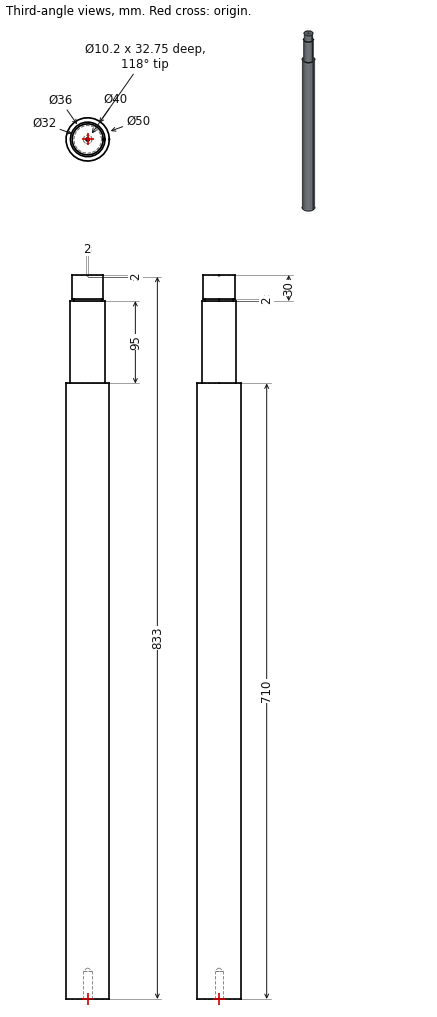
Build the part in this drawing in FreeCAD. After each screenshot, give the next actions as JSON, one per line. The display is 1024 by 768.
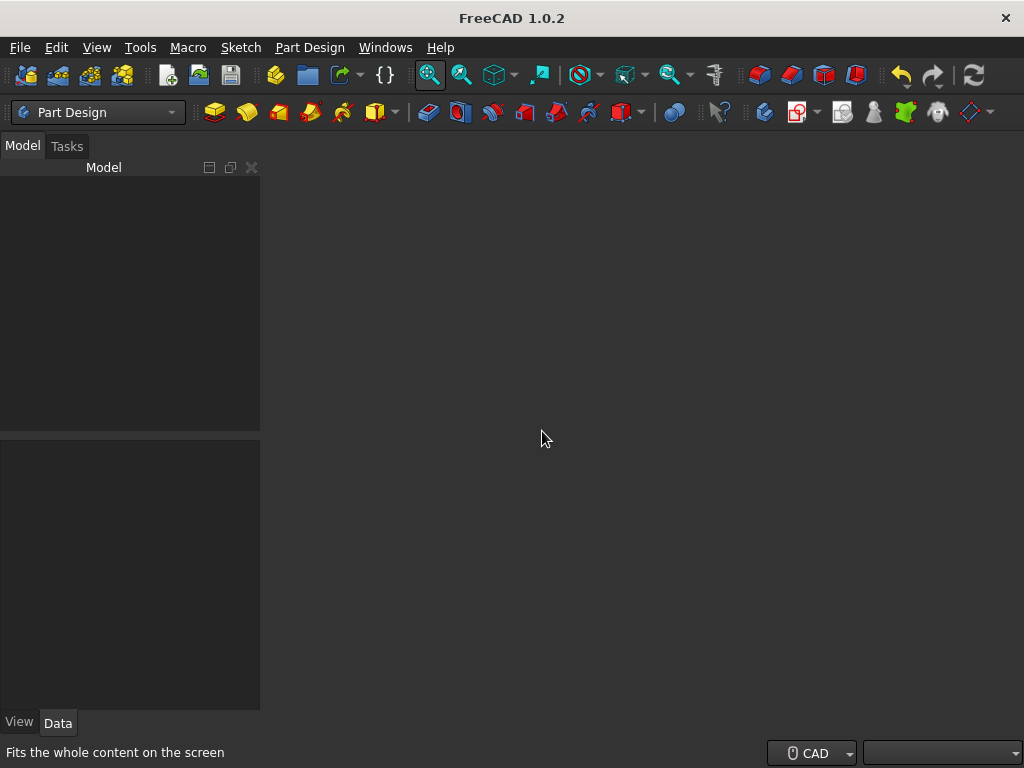
{"action": "left_click", "coordinate": [168, 76]}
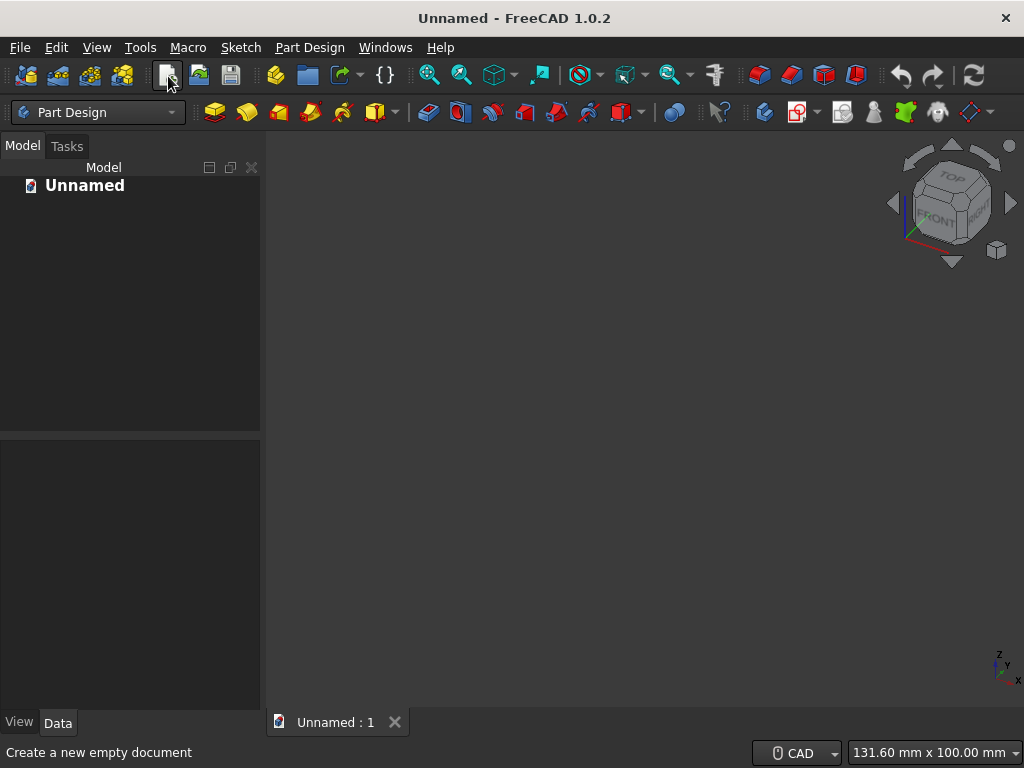
{"action": "left_click", "coordinate": [798, 112]}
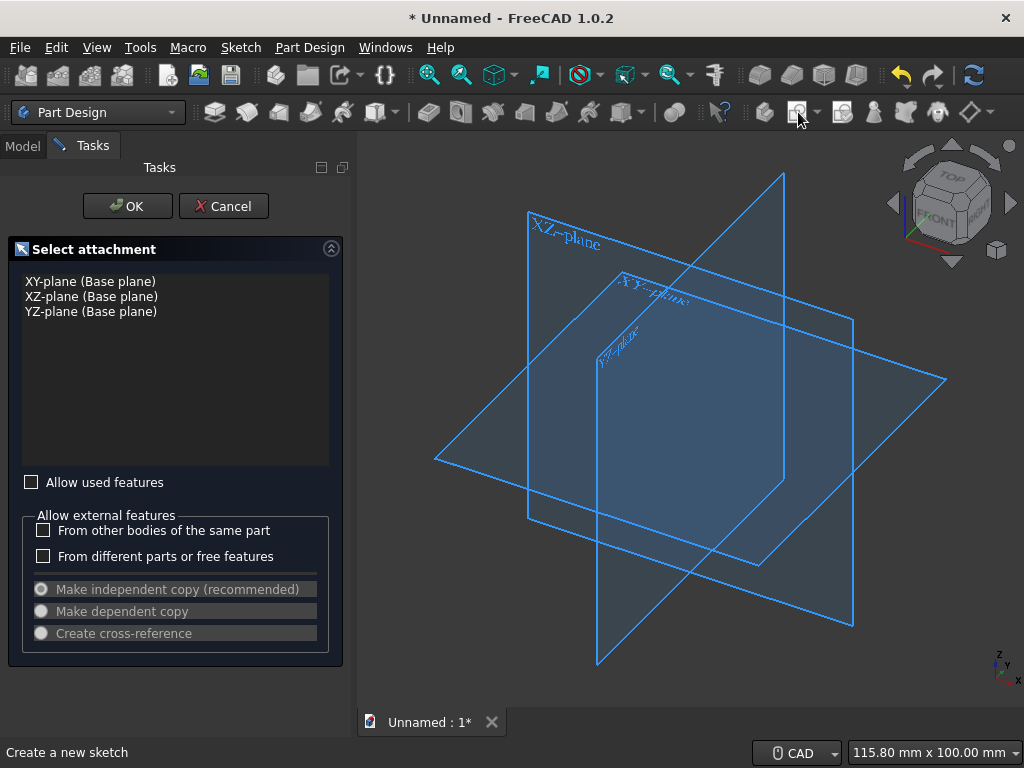
{"action": "left_click", "coordinate": [82, 282]}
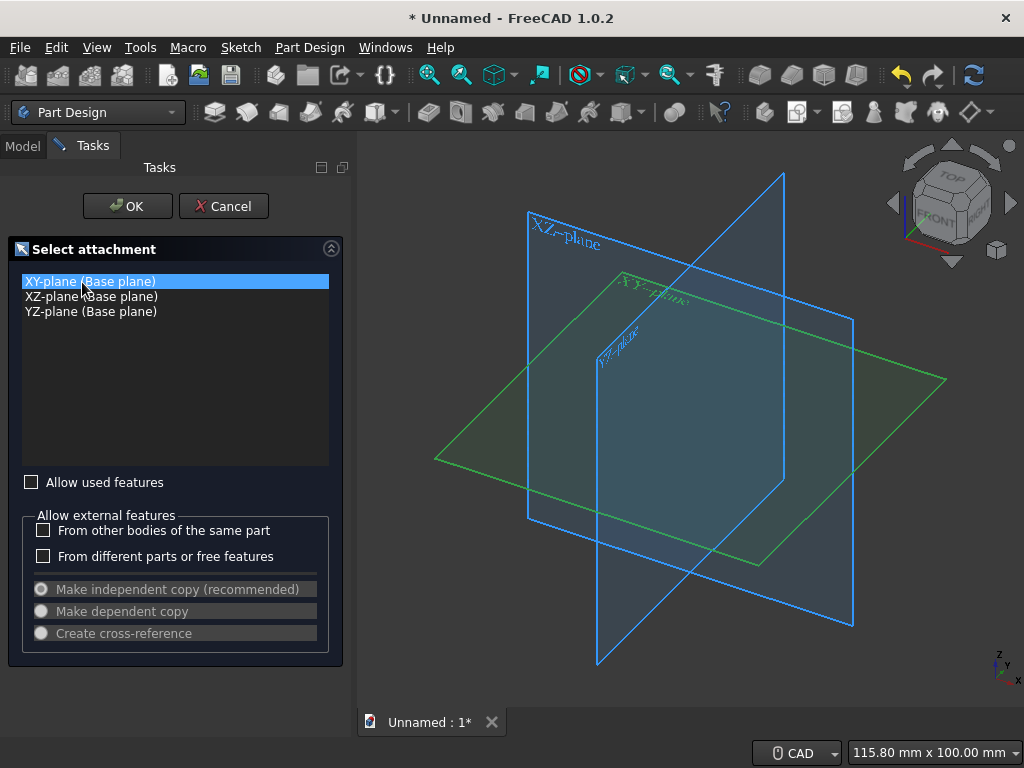
{"action": "left_click", "coordinate": [128, 206]}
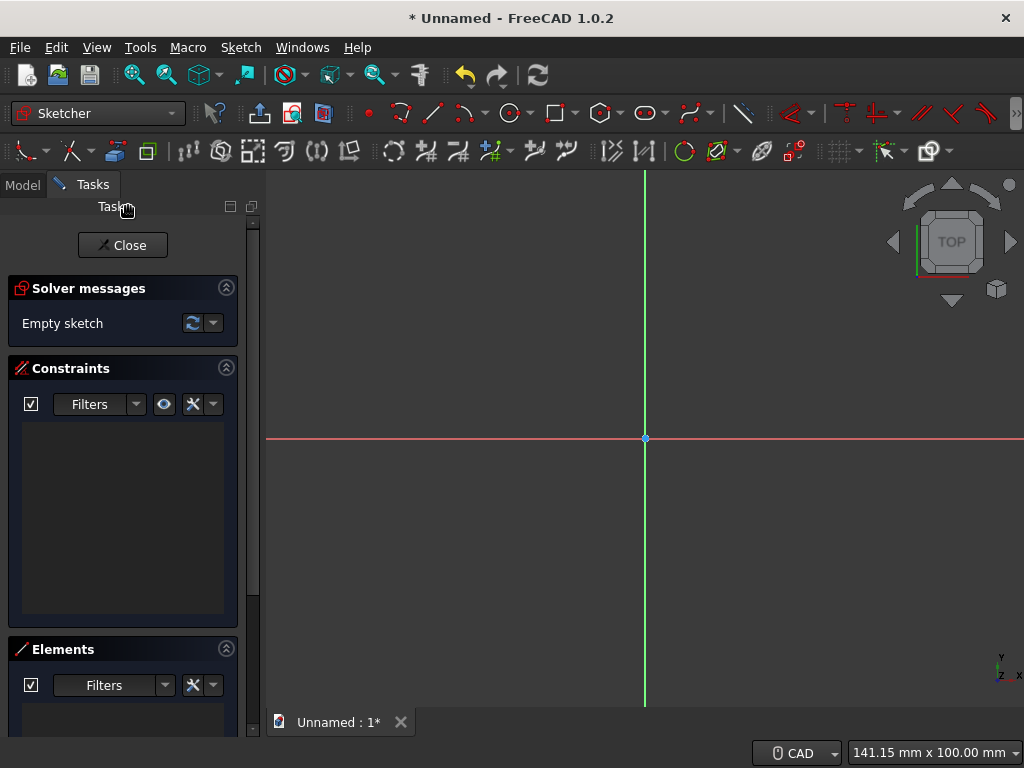
{"action": "left_click", "coordinate": [510, 114]}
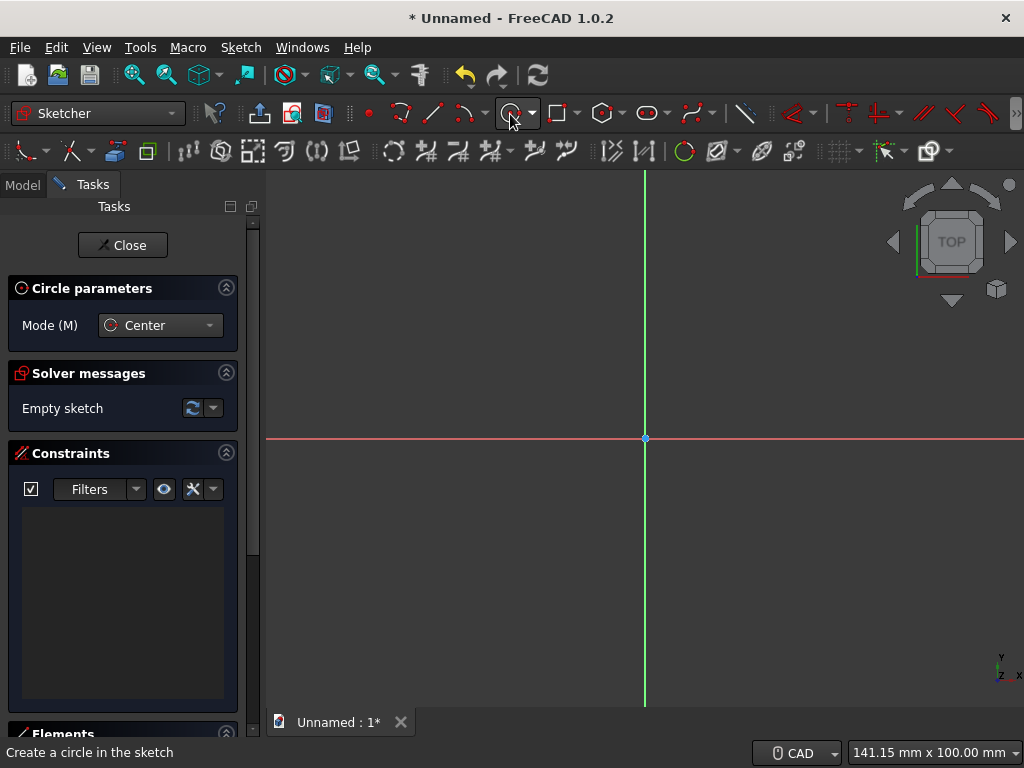
{"action": "left_click", "coordinate": [645, 438]}
{"action": "mouse_move", "coordinate": [740, 344]}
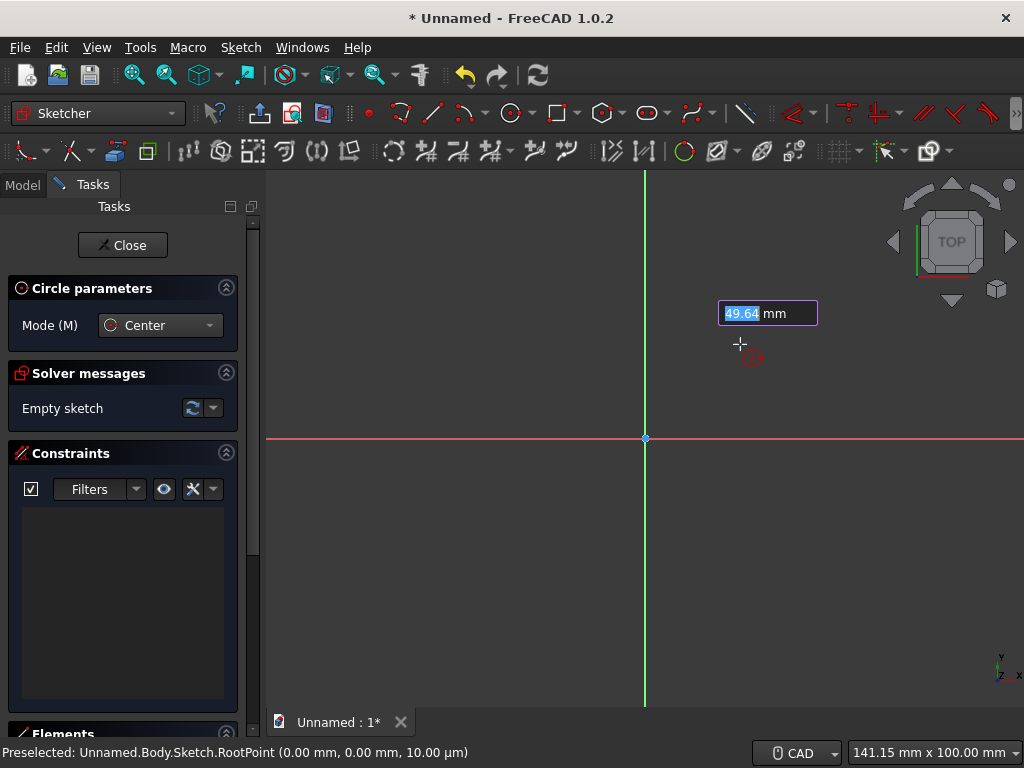
{"action": "type", "text": "50"}
{"action": "key", "text": "Return"}
{"action": "key", "text": "Escape"}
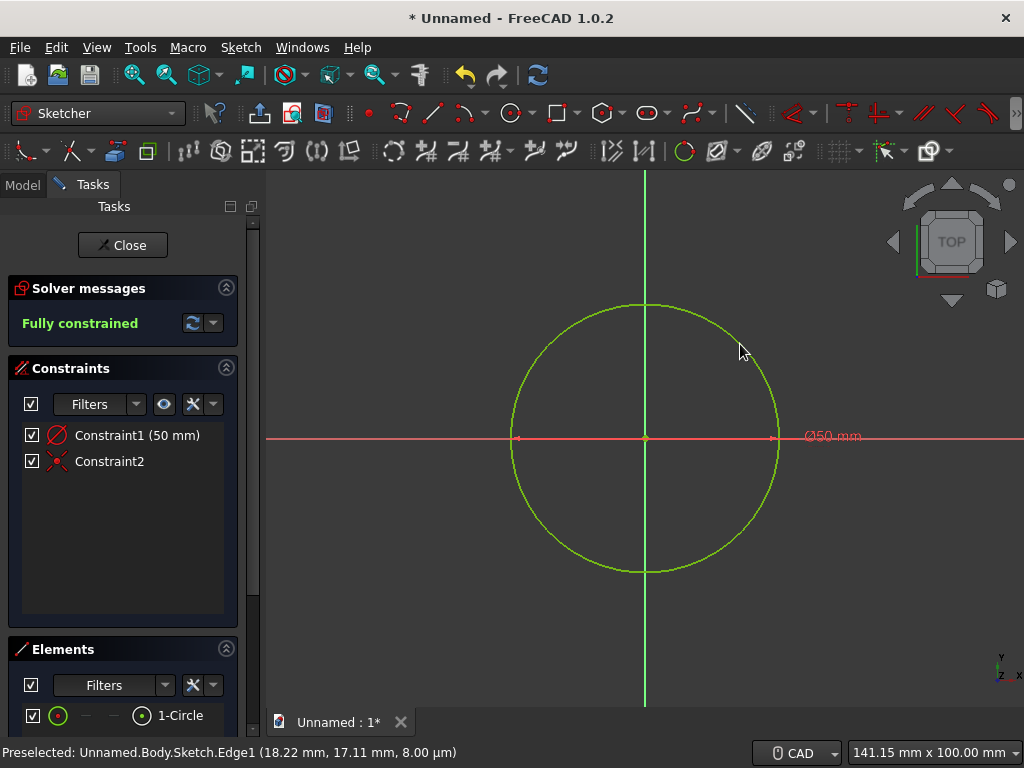
{"action": "left_click", "coordinate": [123, 245]}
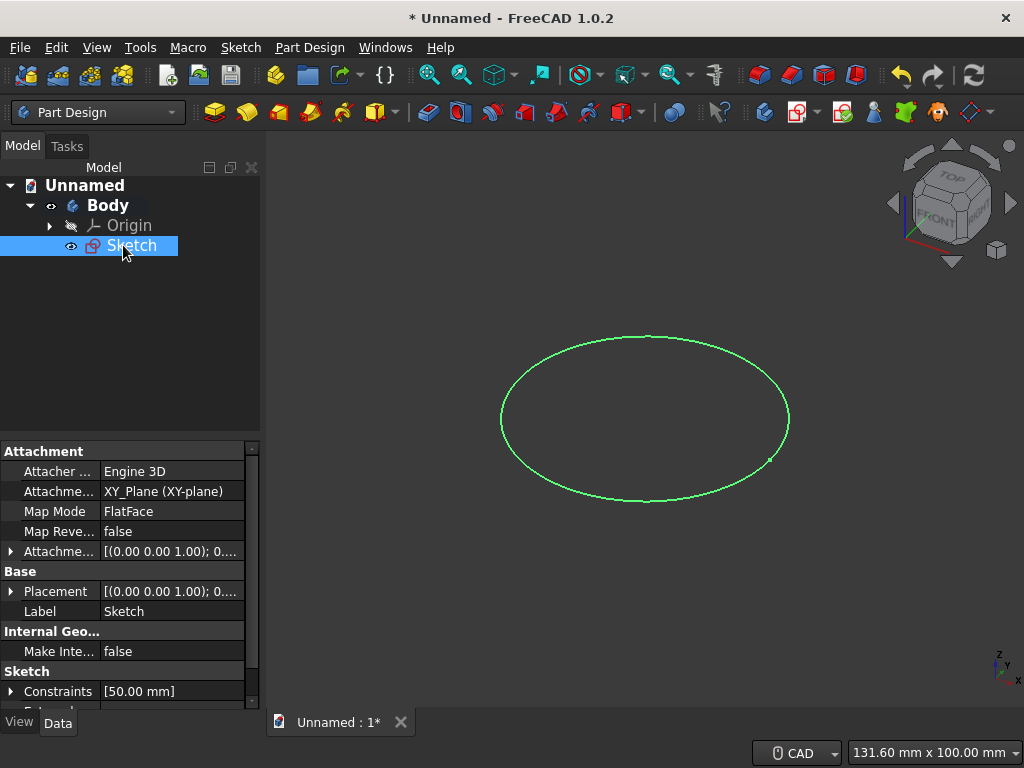
{"action": "left_click", "coordinate": [216, 112]}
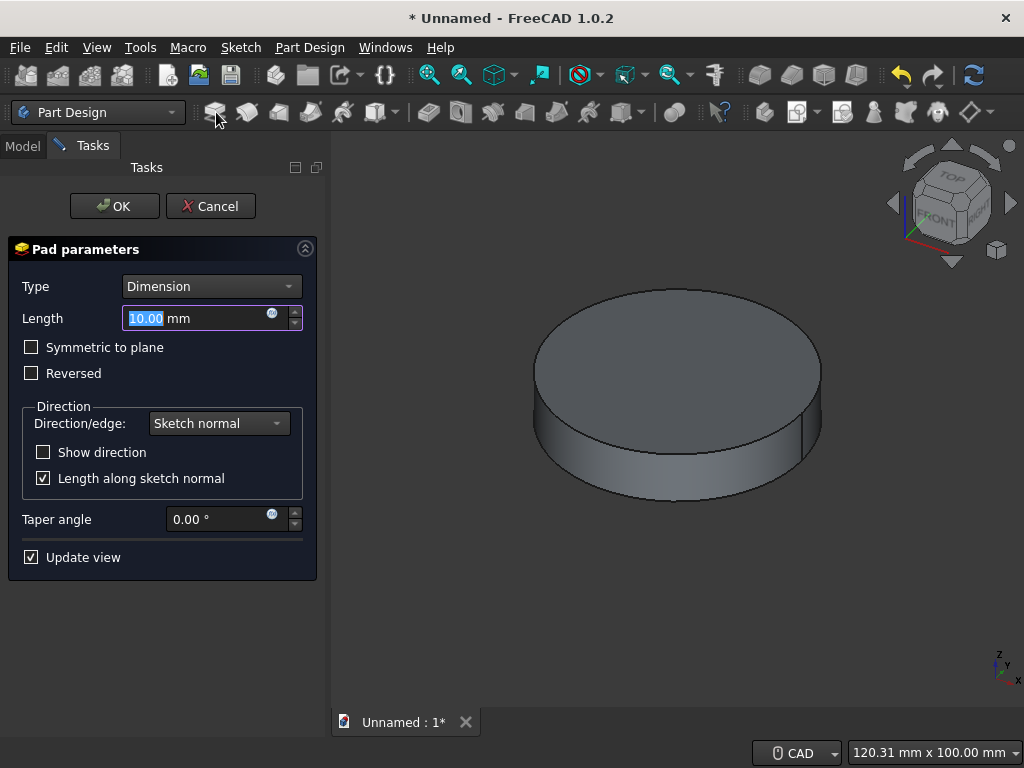
{"action": "type", "text": "710"}
{"action": "key", "text": "Tab"}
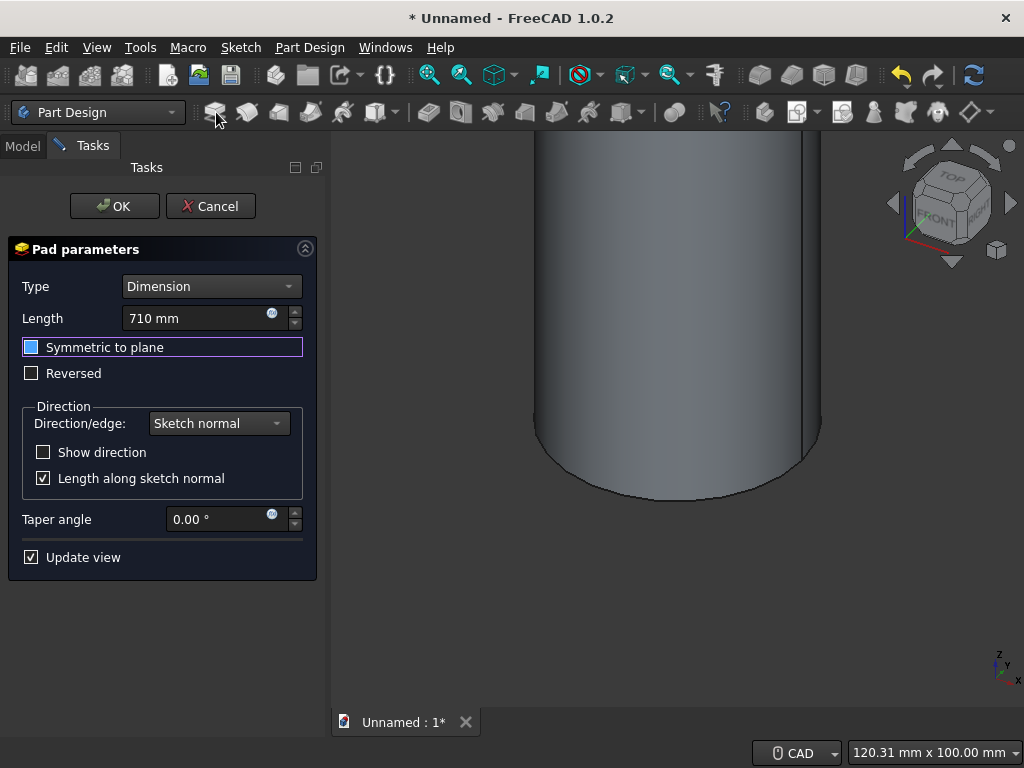
{"action": "left_click", "coordinate": [115, 206]}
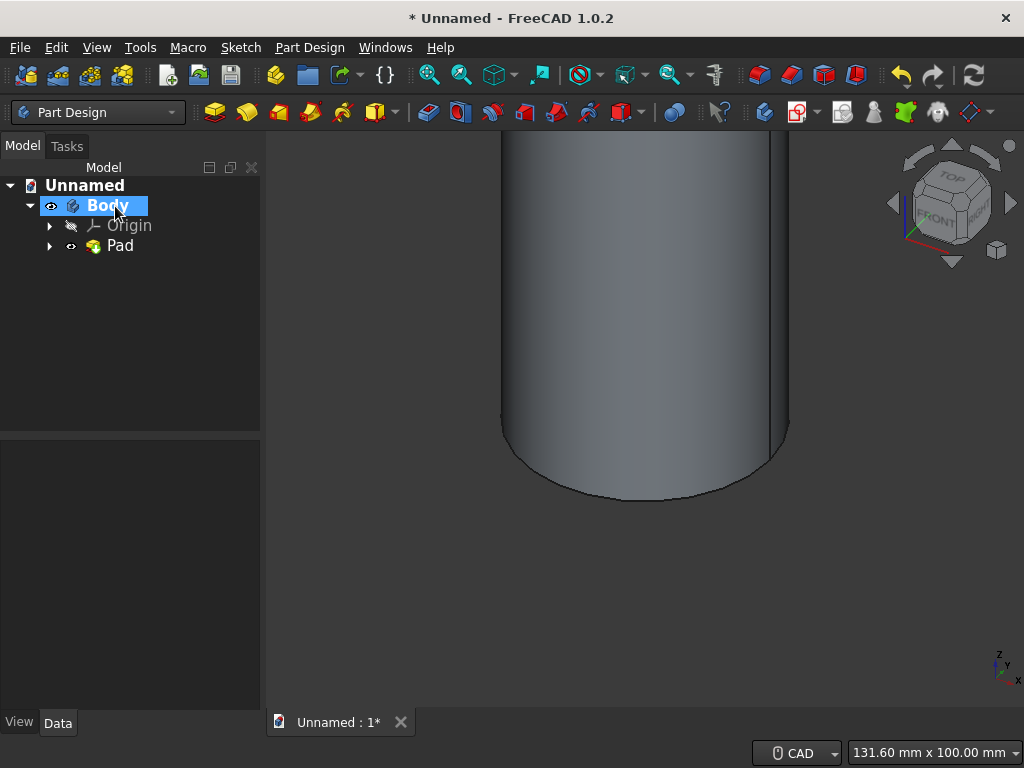
{"action": "left_click", "coordinate": [430, 76]}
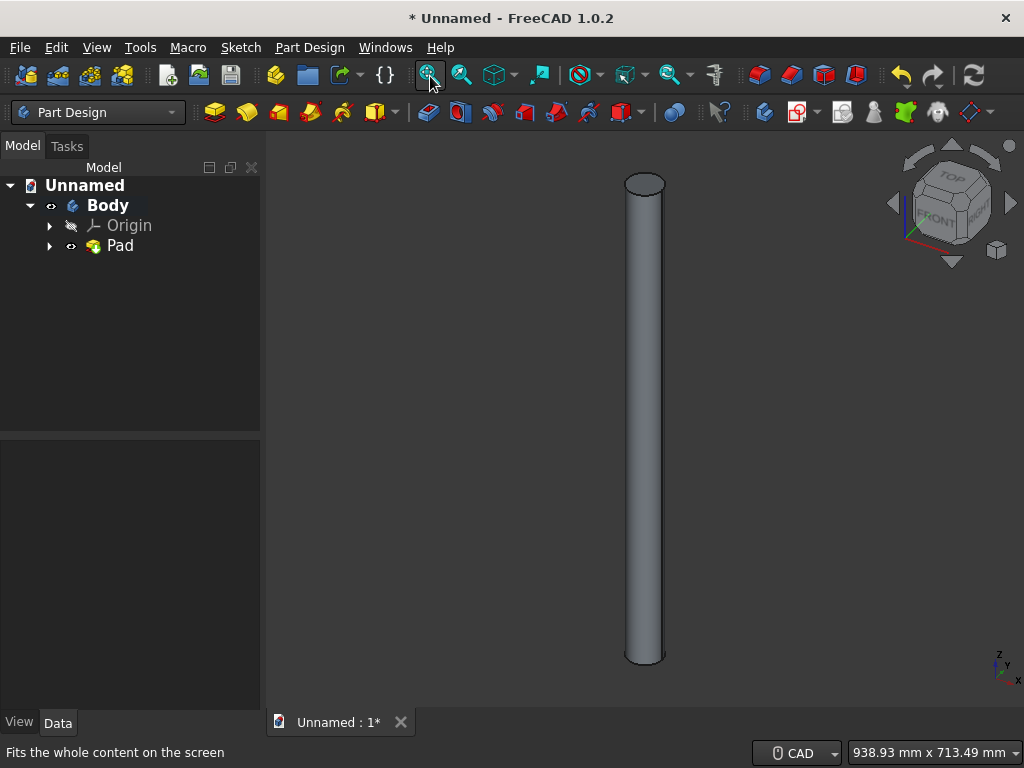
{"action": "left_click", "coordinate": [645, 183]}